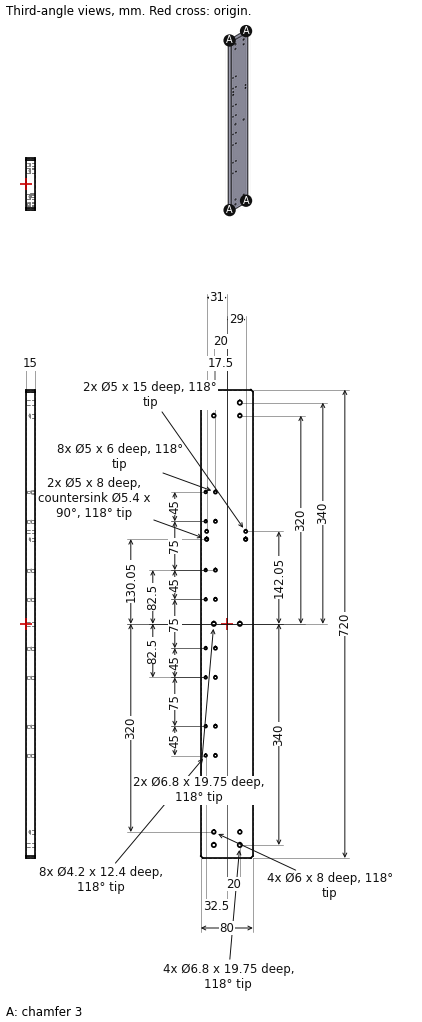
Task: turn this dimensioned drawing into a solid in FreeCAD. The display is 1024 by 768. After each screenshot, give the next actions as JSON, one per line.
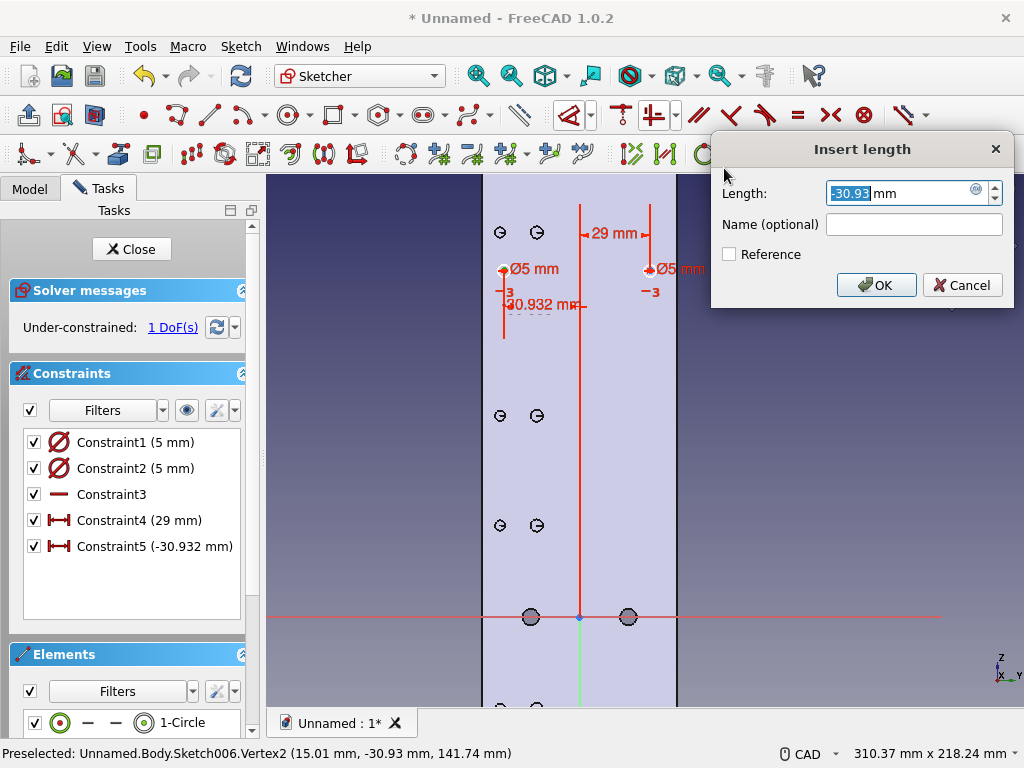
{"action": "type", "text": "-31"}
{"action": "key", "text": "Return"}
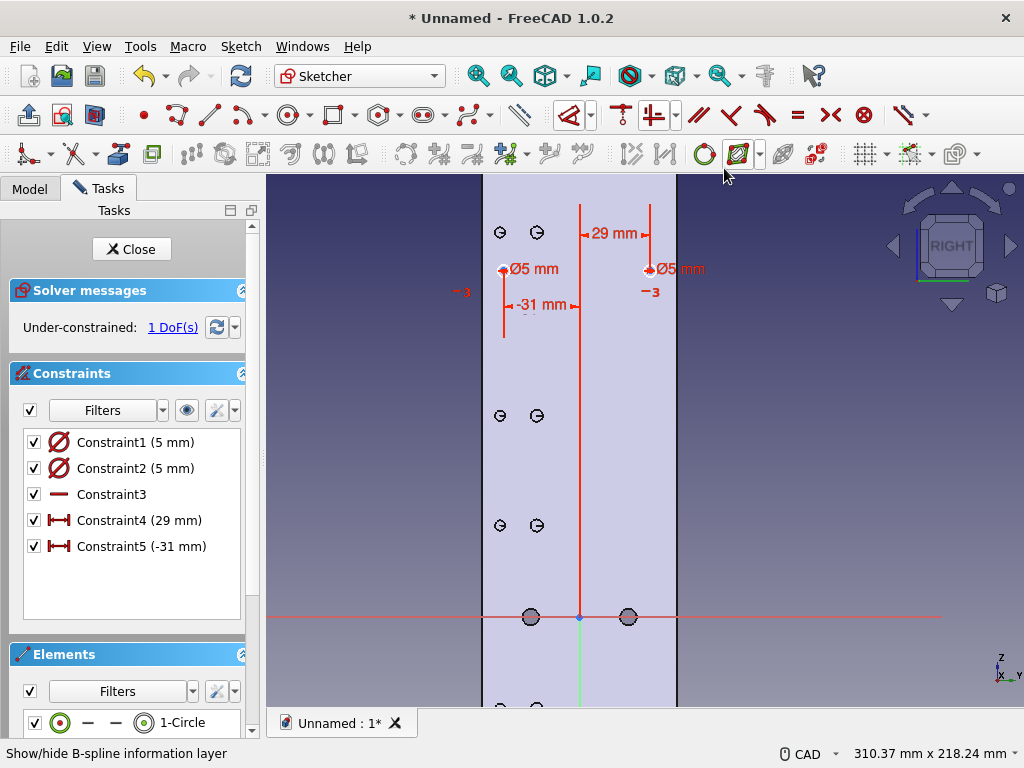
{"action": "left_click", "coordinate": [650, 271]}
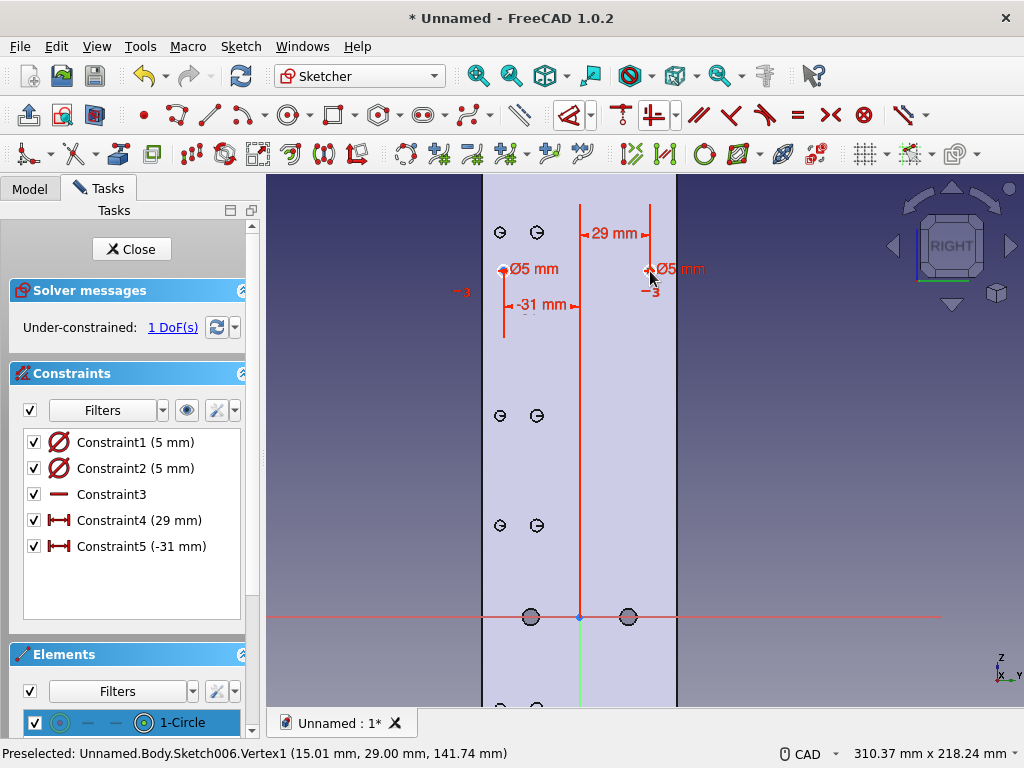
{"action": "key", "text": "i"}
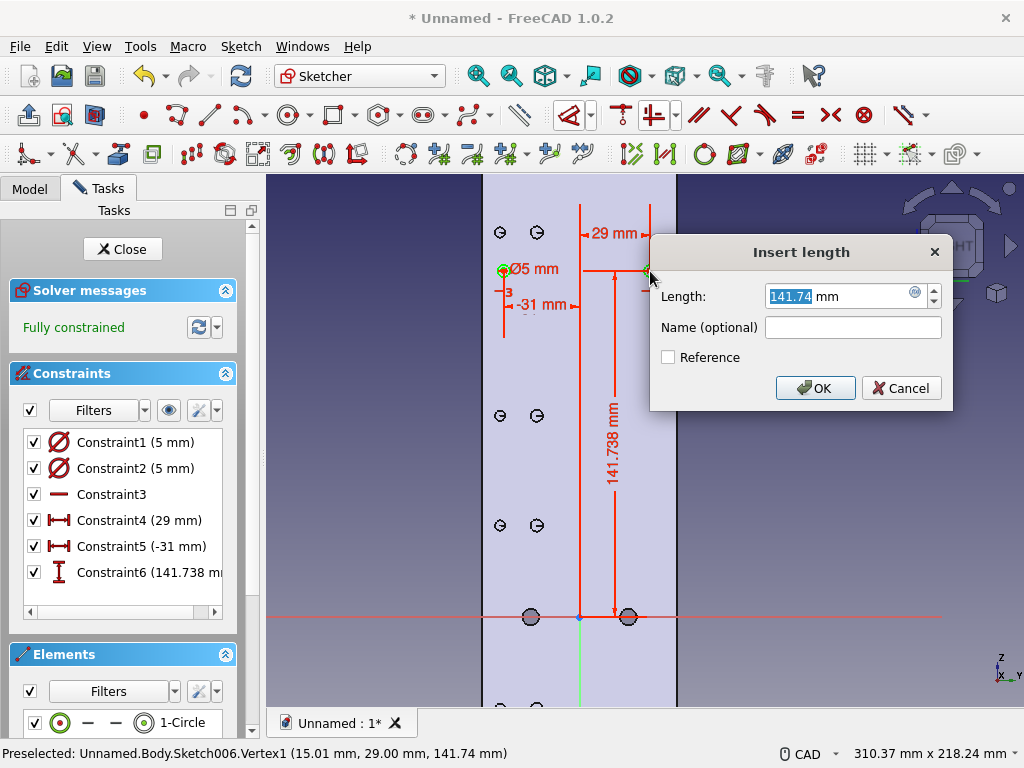
{"action": "type", "text": "142.05"}
{"action": "key", "text": "Return"}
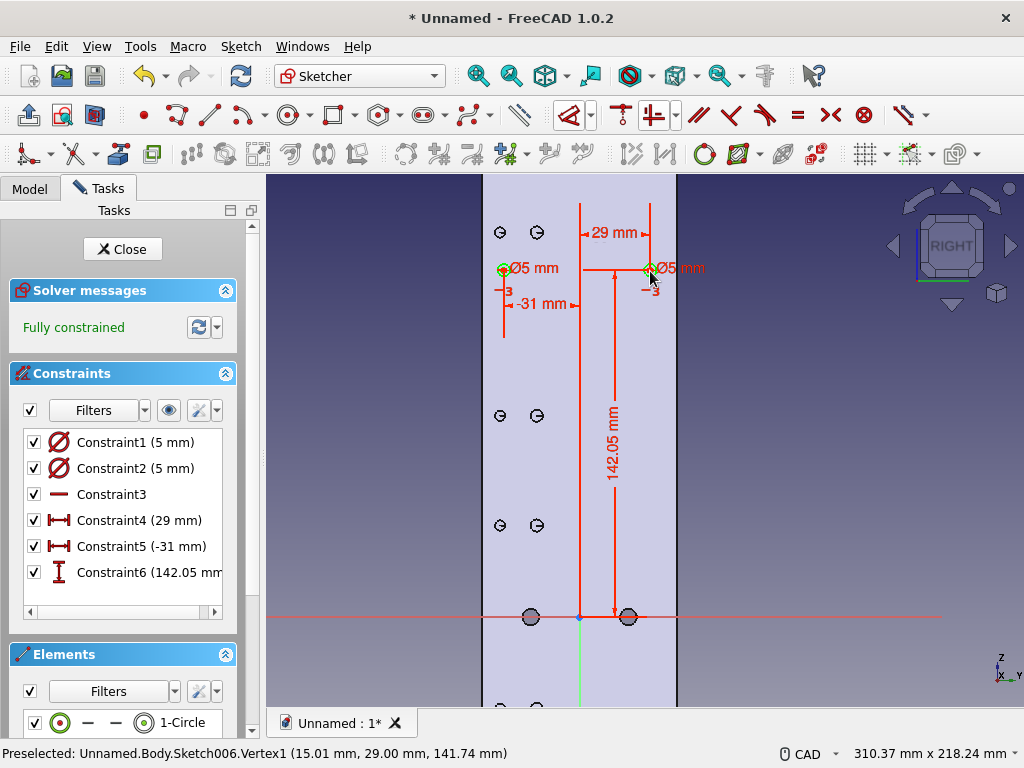
{"action": "left_click", "coordinate": [123, 249]}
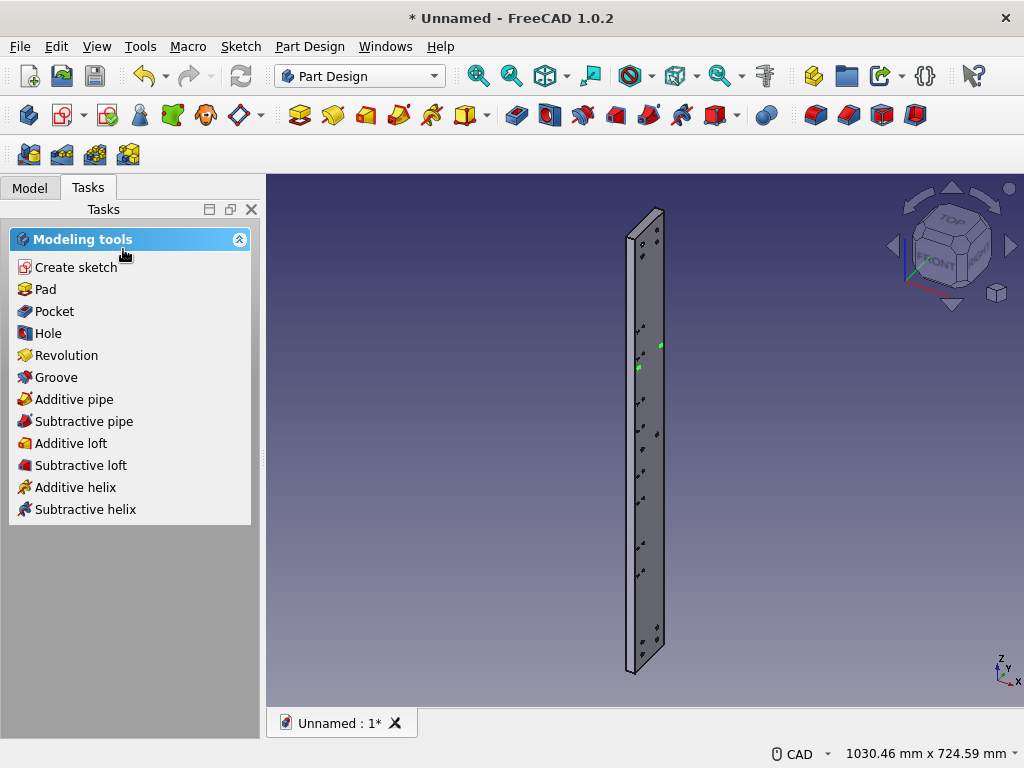
{"action": "left_click", "coordinate": [550, 116]}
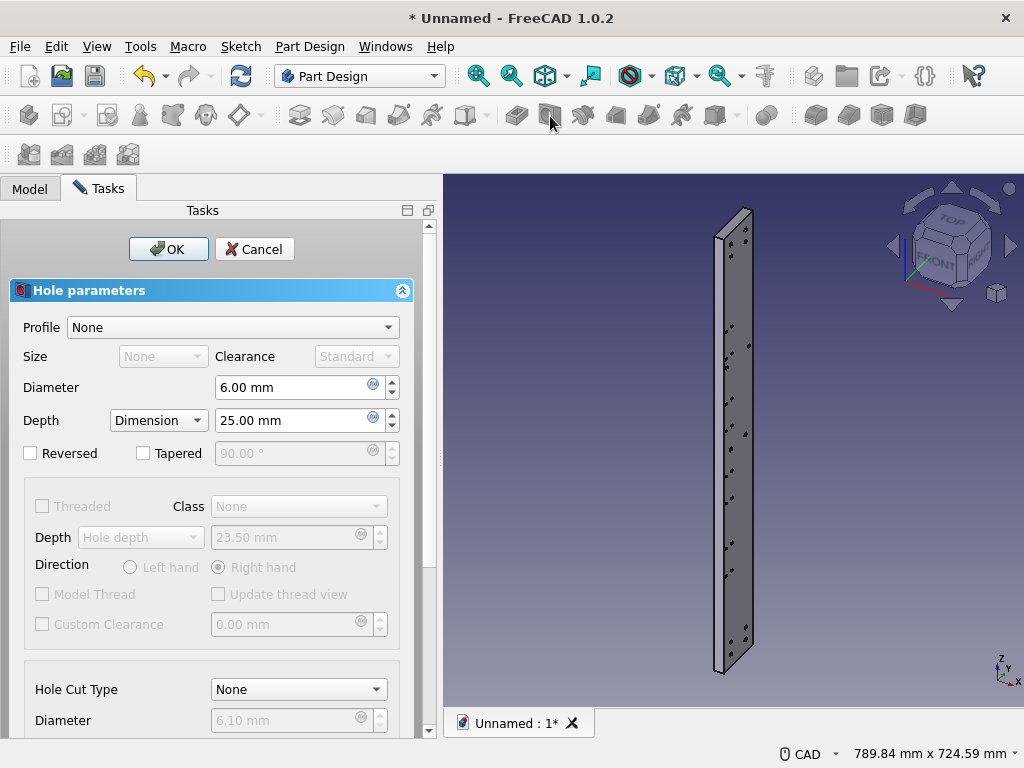
{"action": "triple_click", "coordinate": [300, 388]}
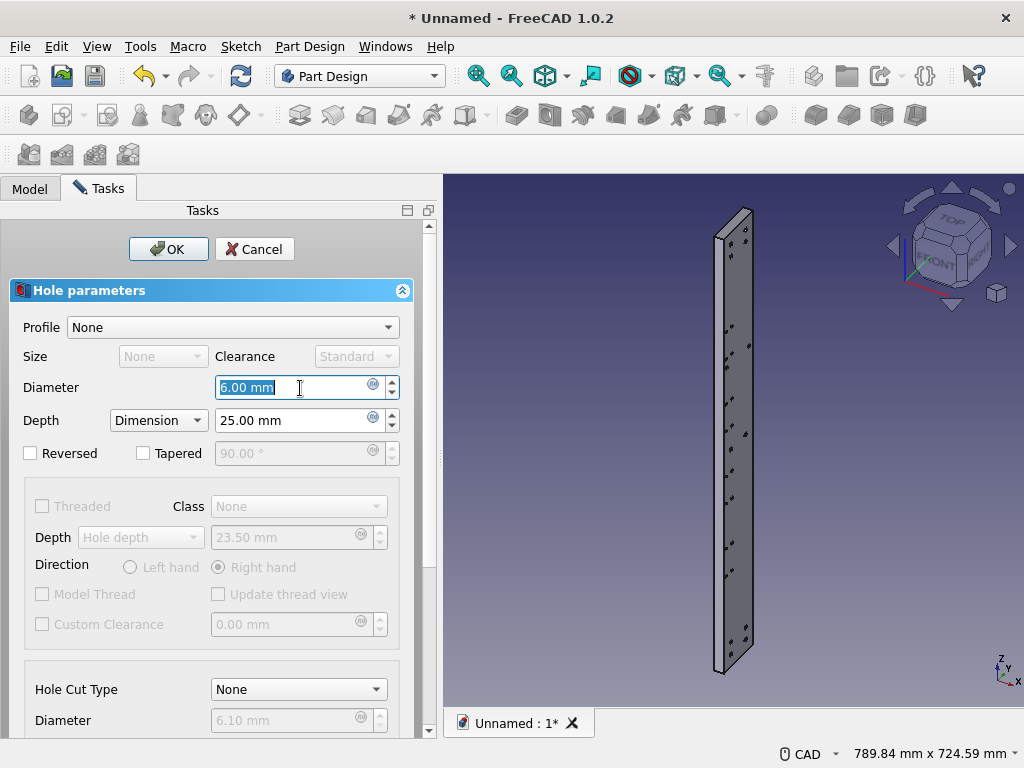
{"action": "type", "text": "5"}
{"action": "key", "text": "Tab"}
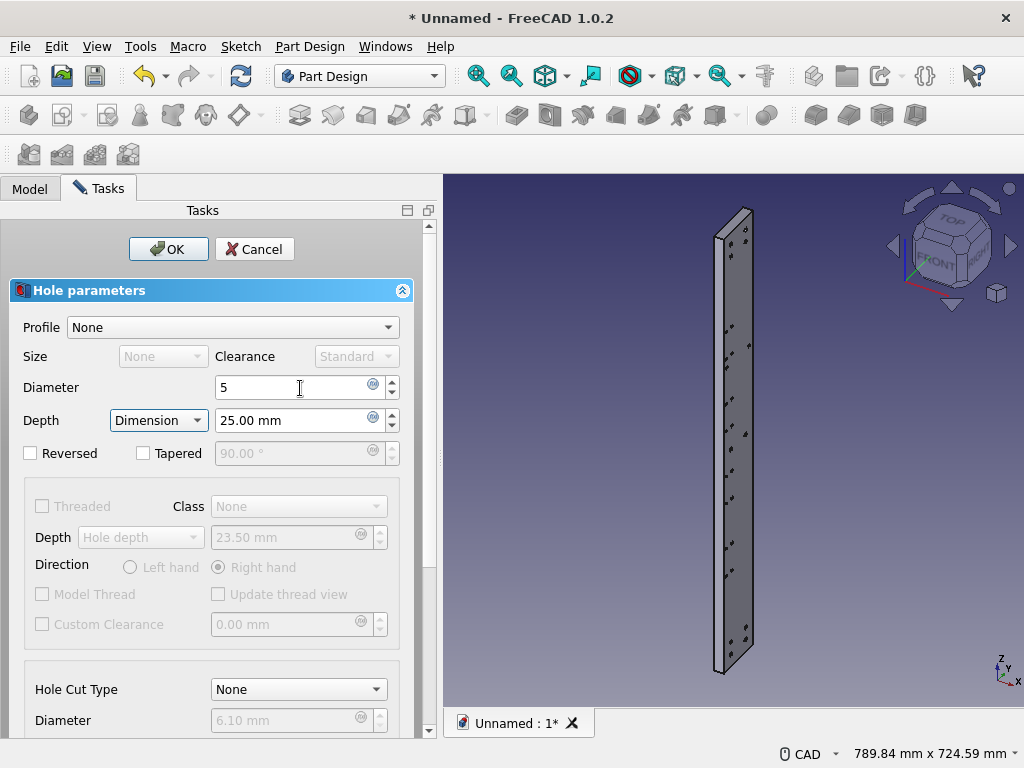
{"action": "triple_click", "coordinate": [300, 420]}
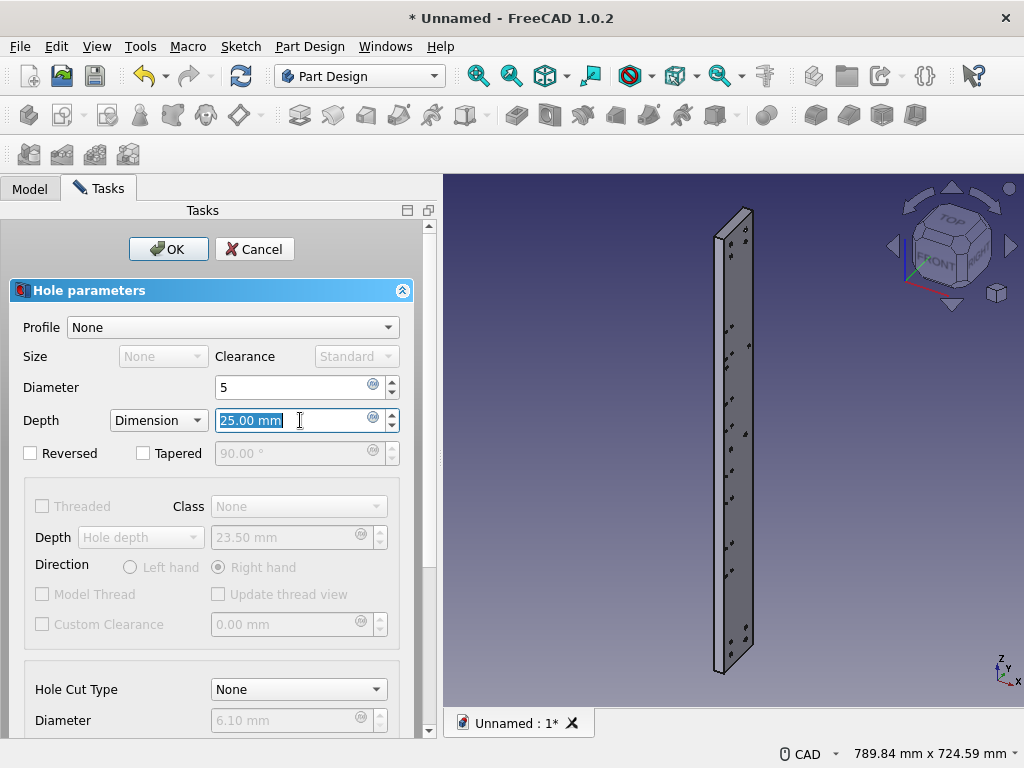
{"action": "type", "text": "15"}
{"action": "key", "text": "Tab"}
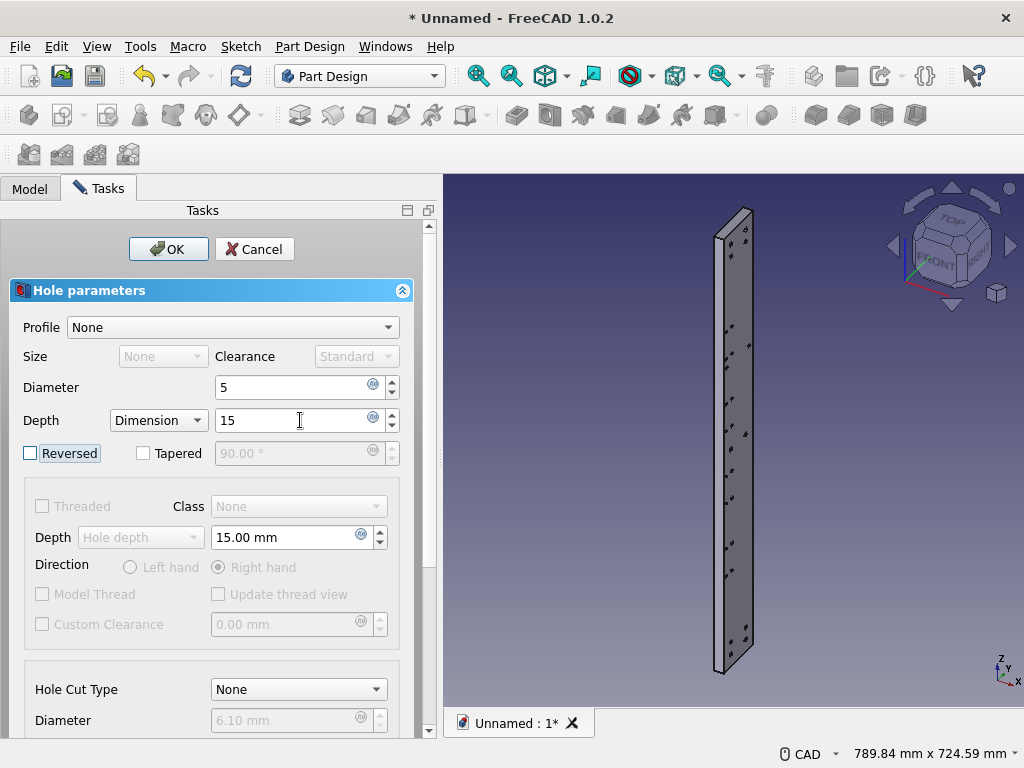
{"action": "left_click", "coordinate": [169, 249]}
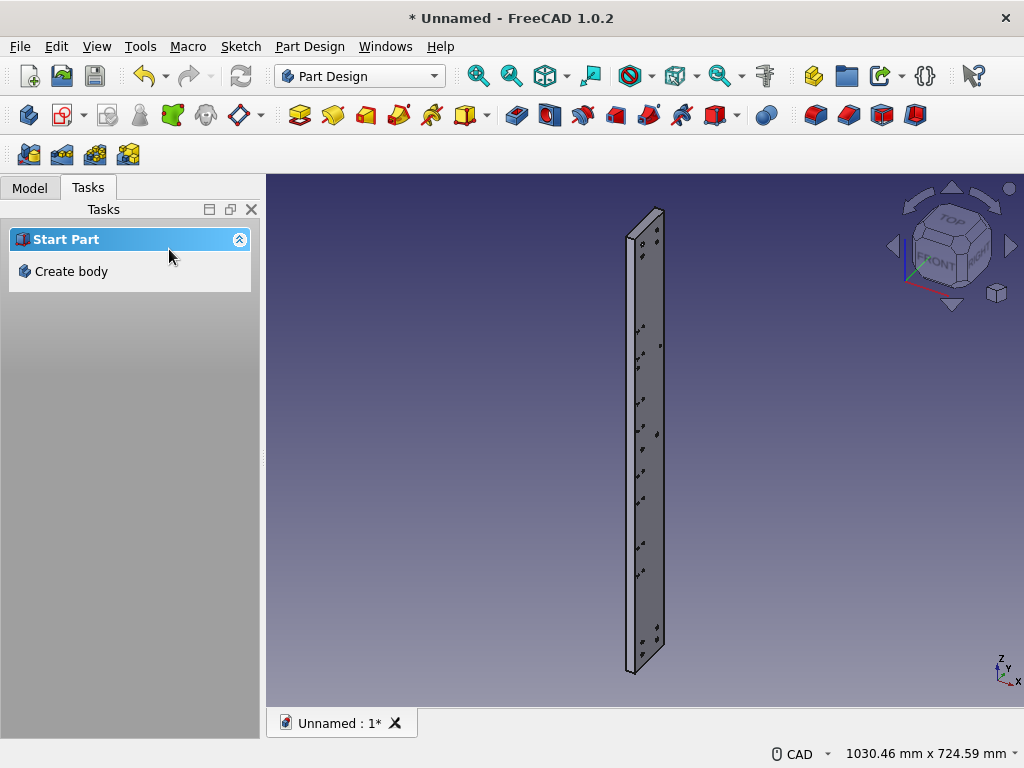
{"action": "left_click", "coordinate": [654, 375]}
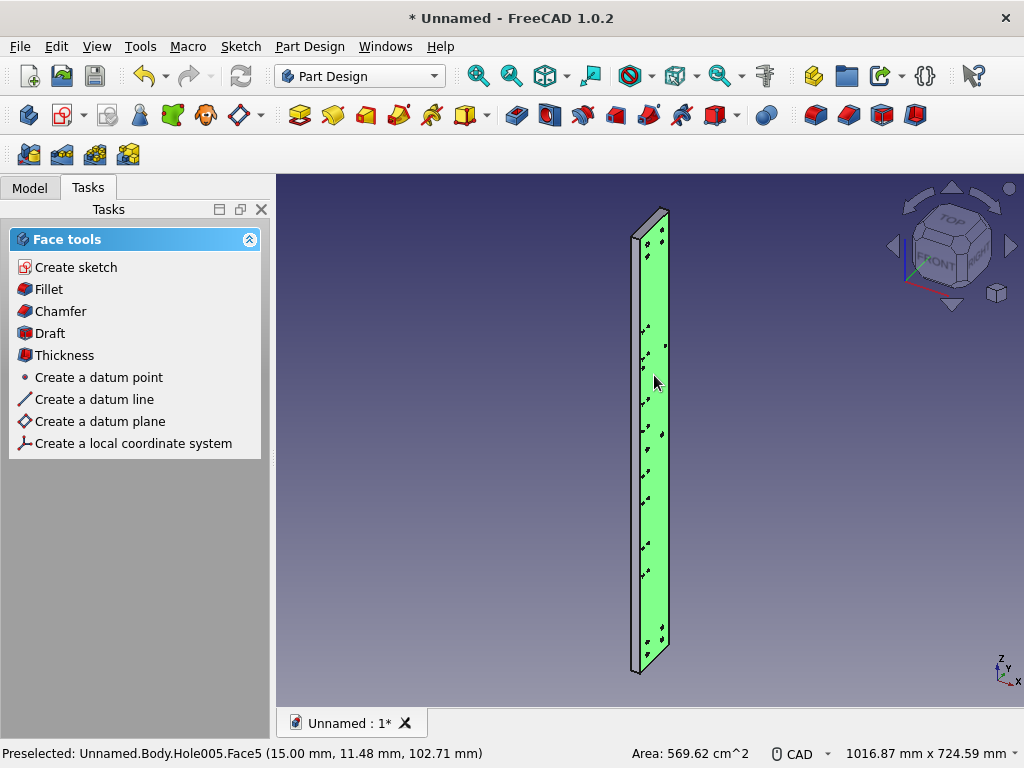
{"action": "left_click", "coordinate": [62, 116]}